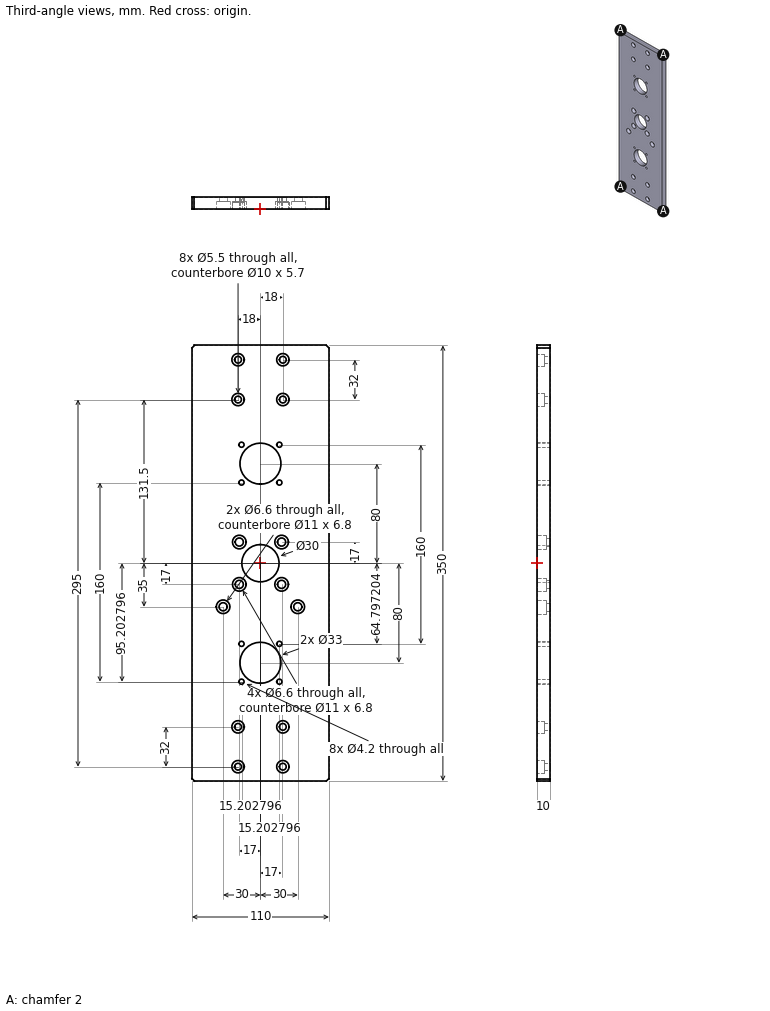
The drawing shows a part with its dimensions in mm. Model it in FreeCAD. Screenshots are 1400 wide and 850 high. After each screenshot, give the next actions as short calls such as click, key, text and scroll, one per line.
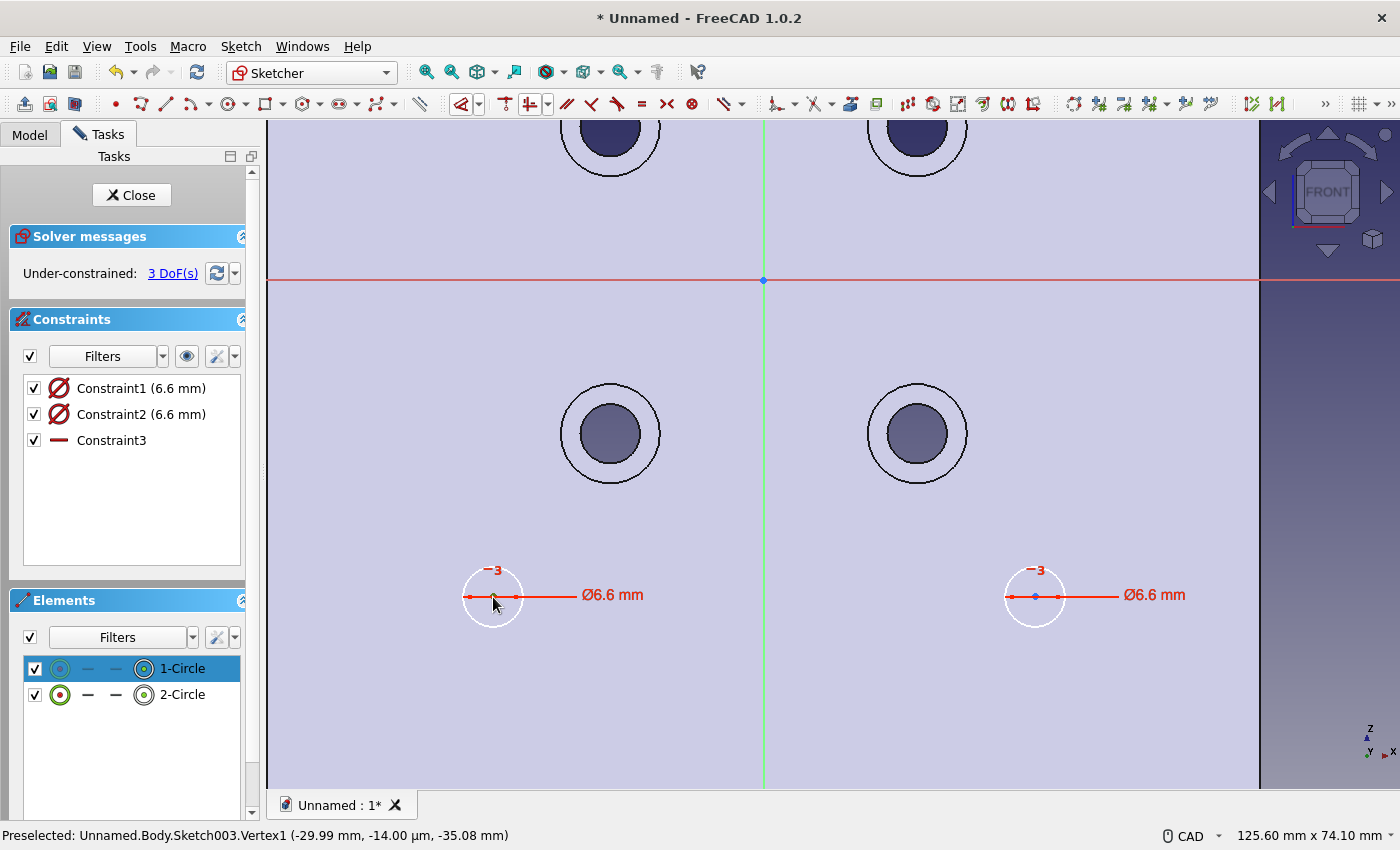
key(l)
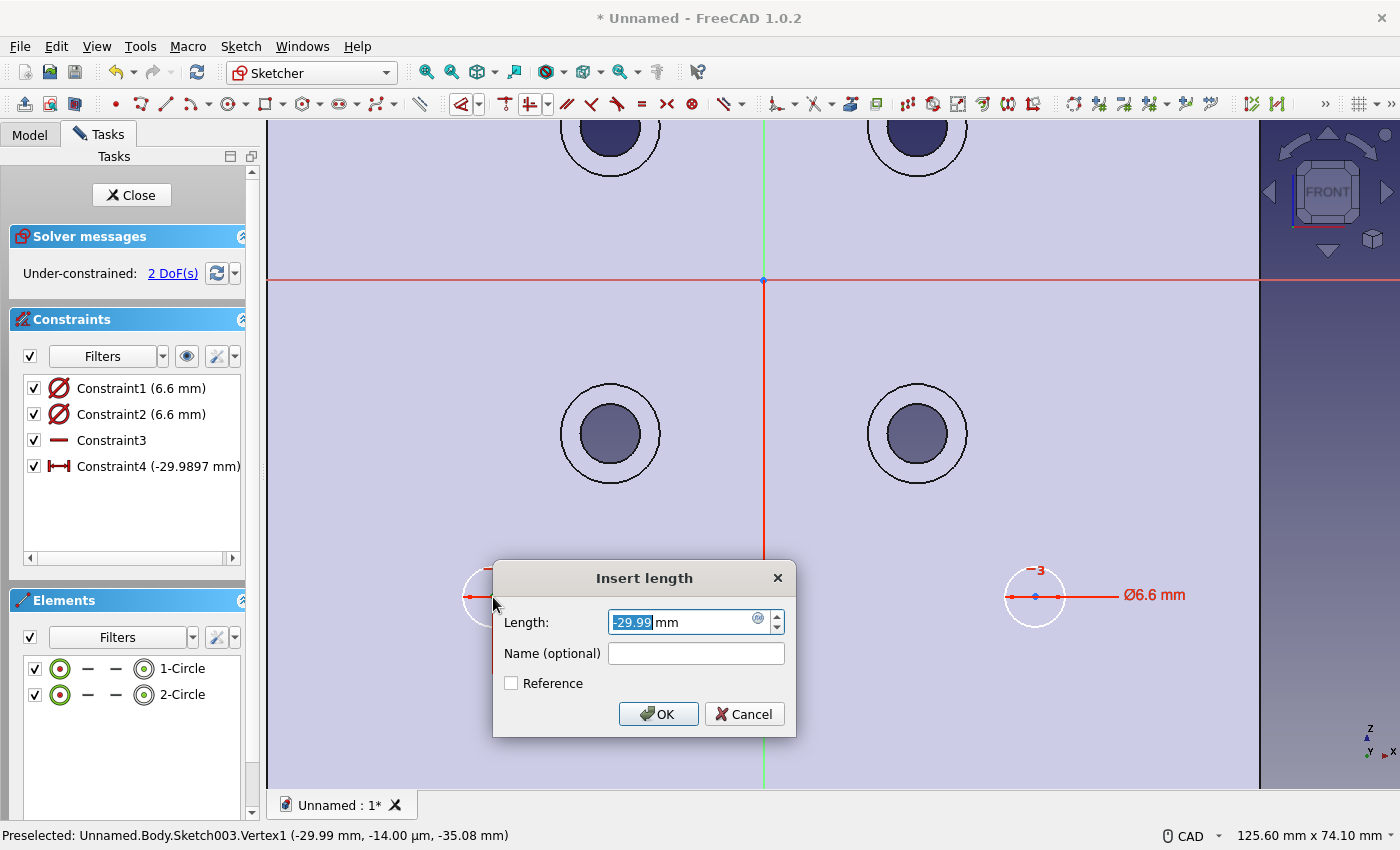
text(-30)
key(Return)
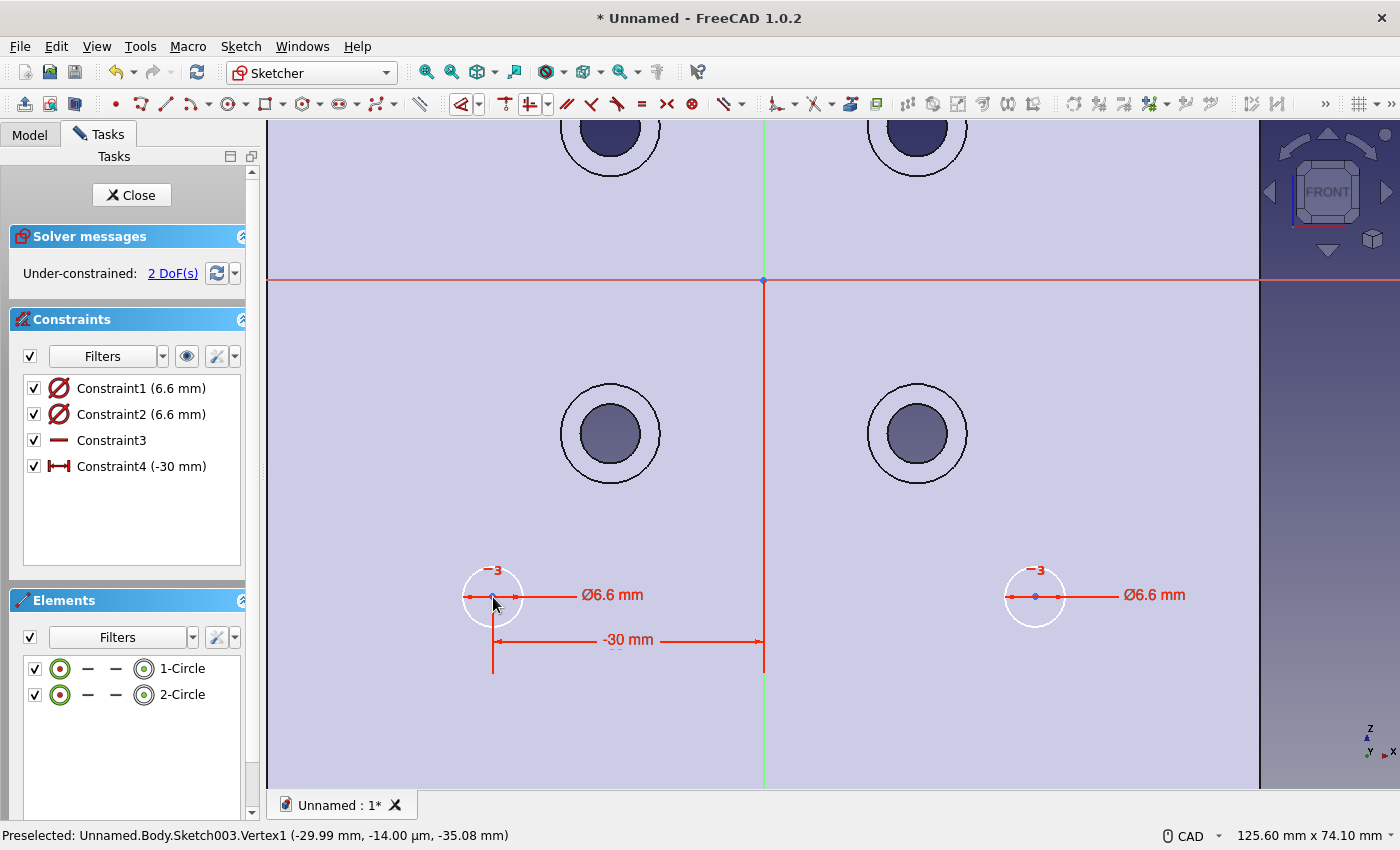
click(493, 597)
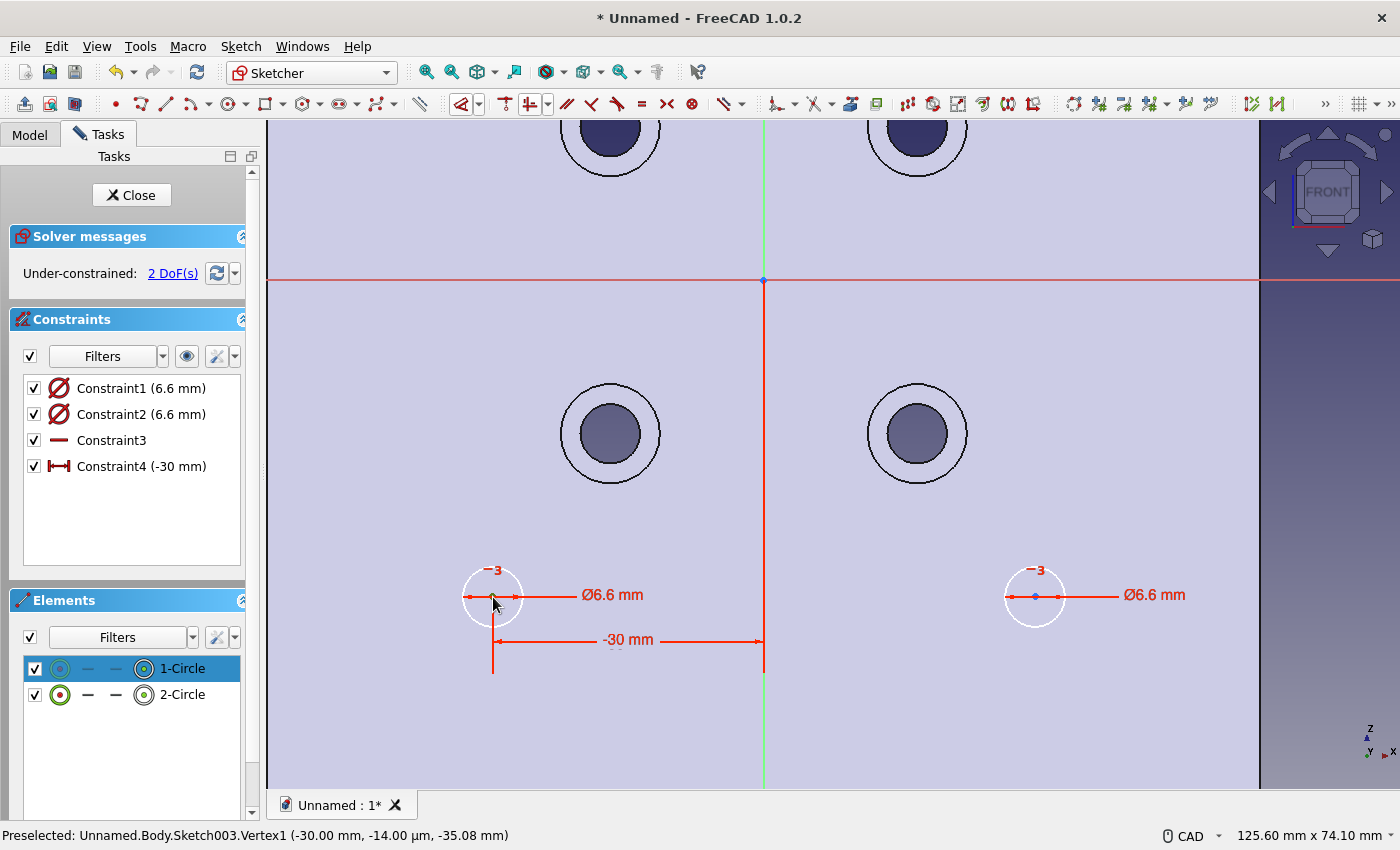
click(478, 104)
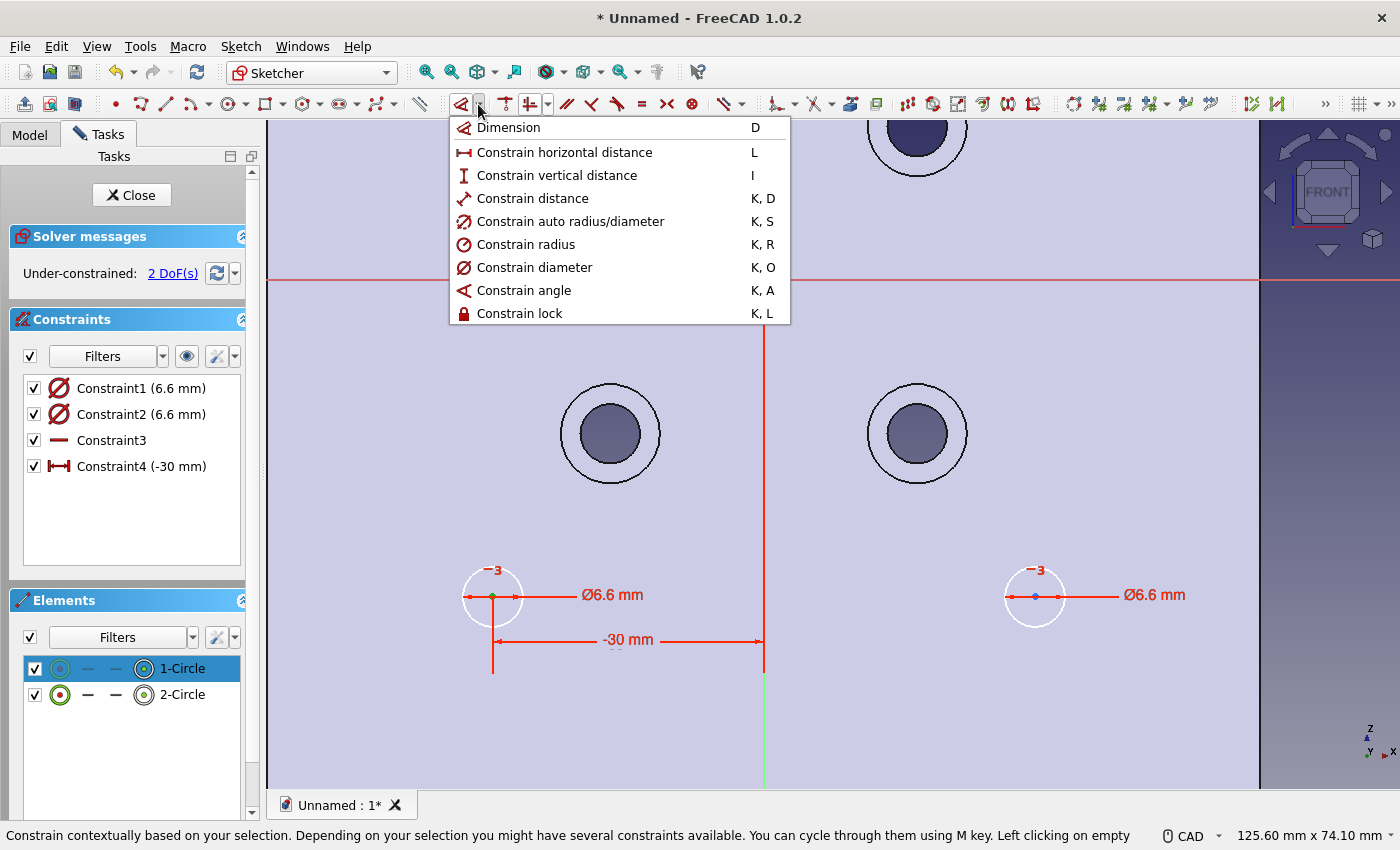
click(620, 176)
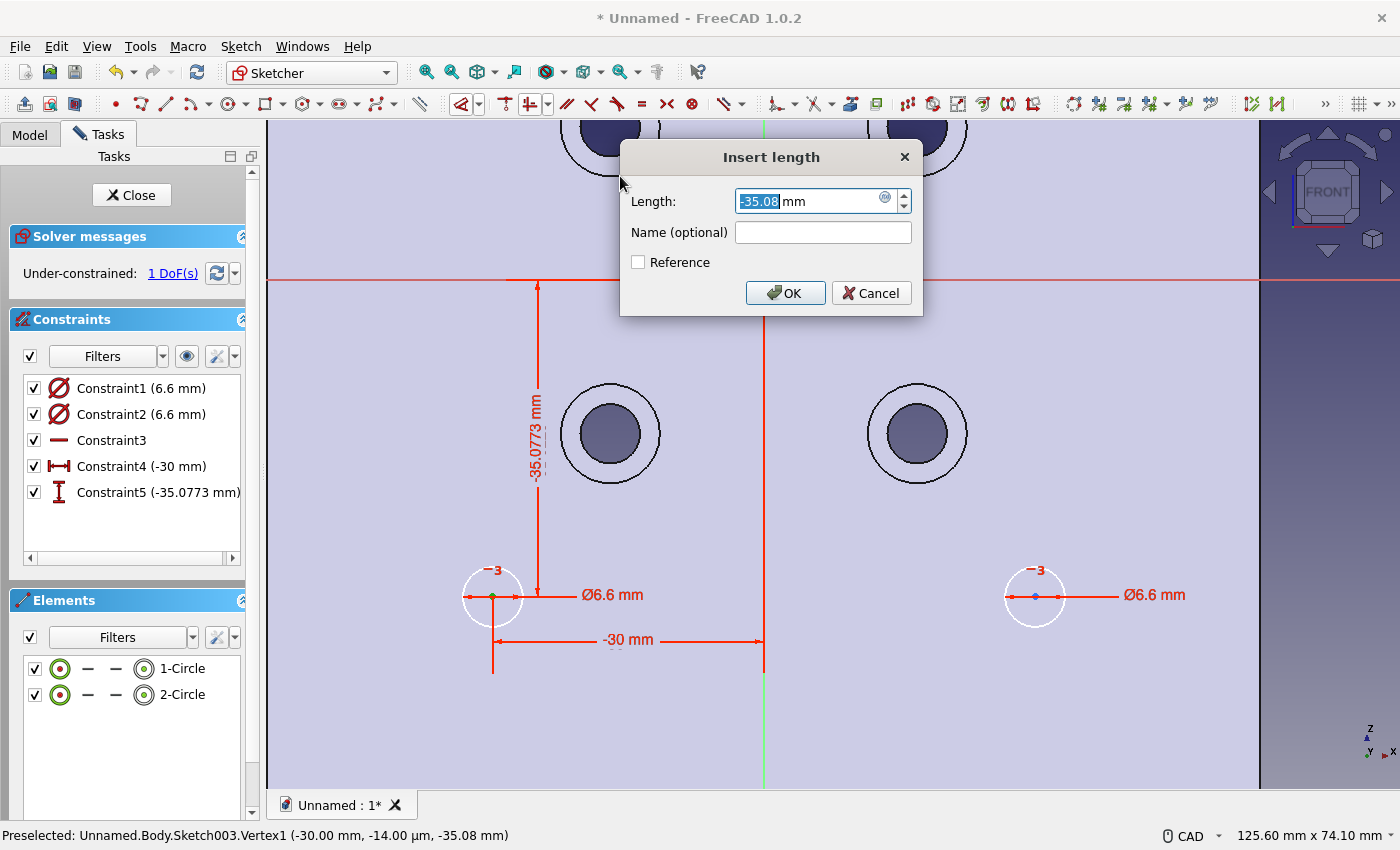
text(-35)
key(Return)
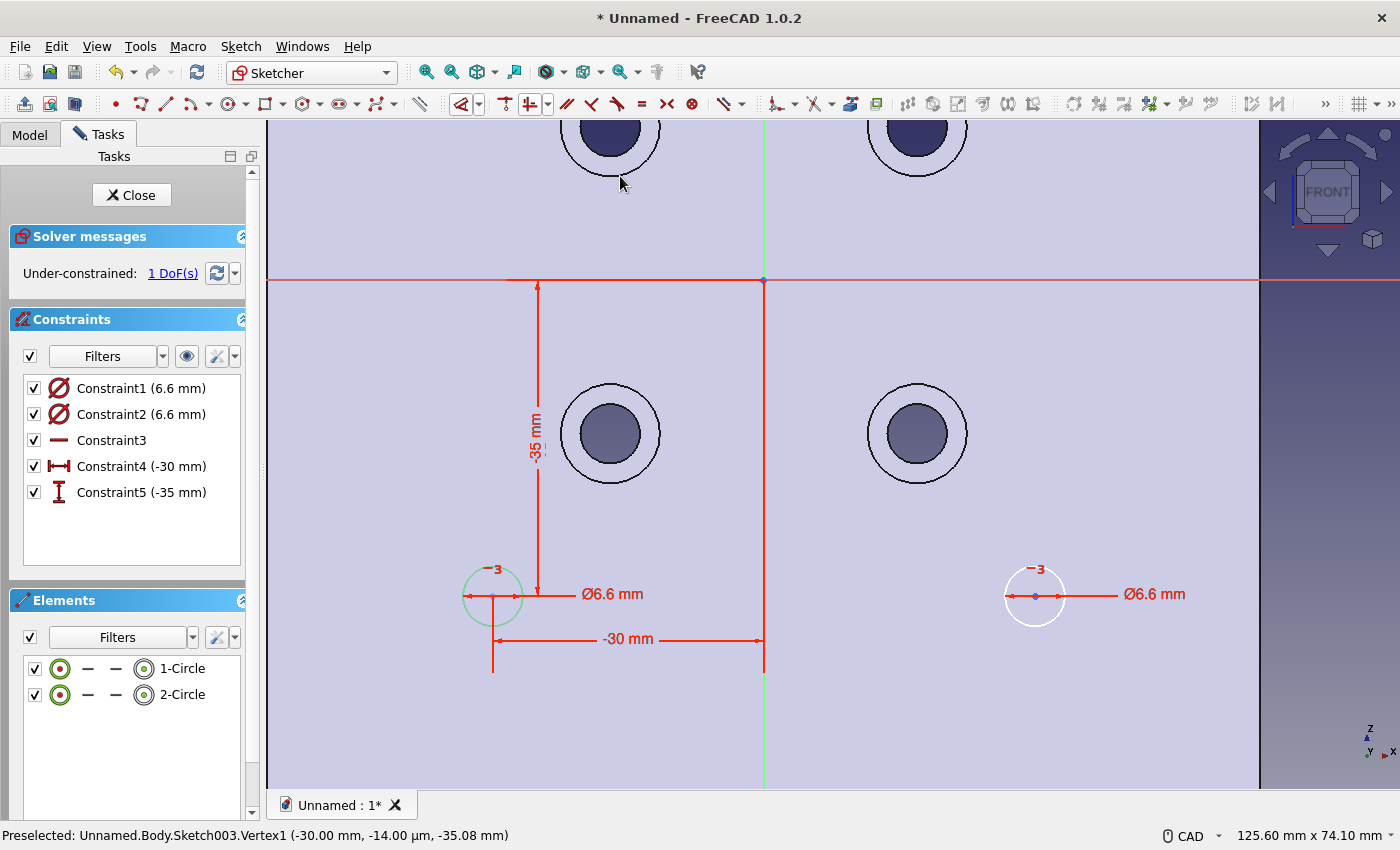
click(1035, 596)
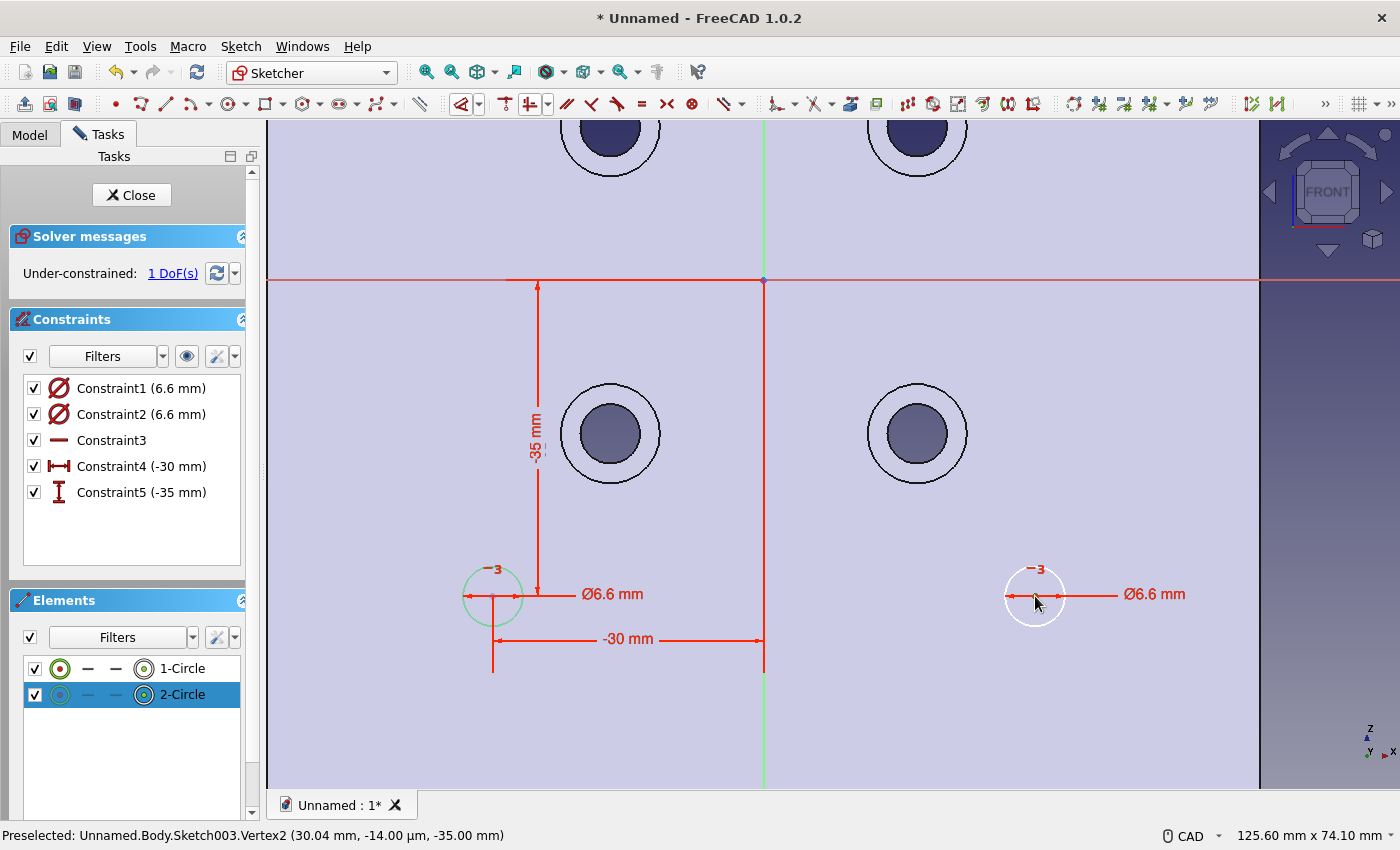
key(l)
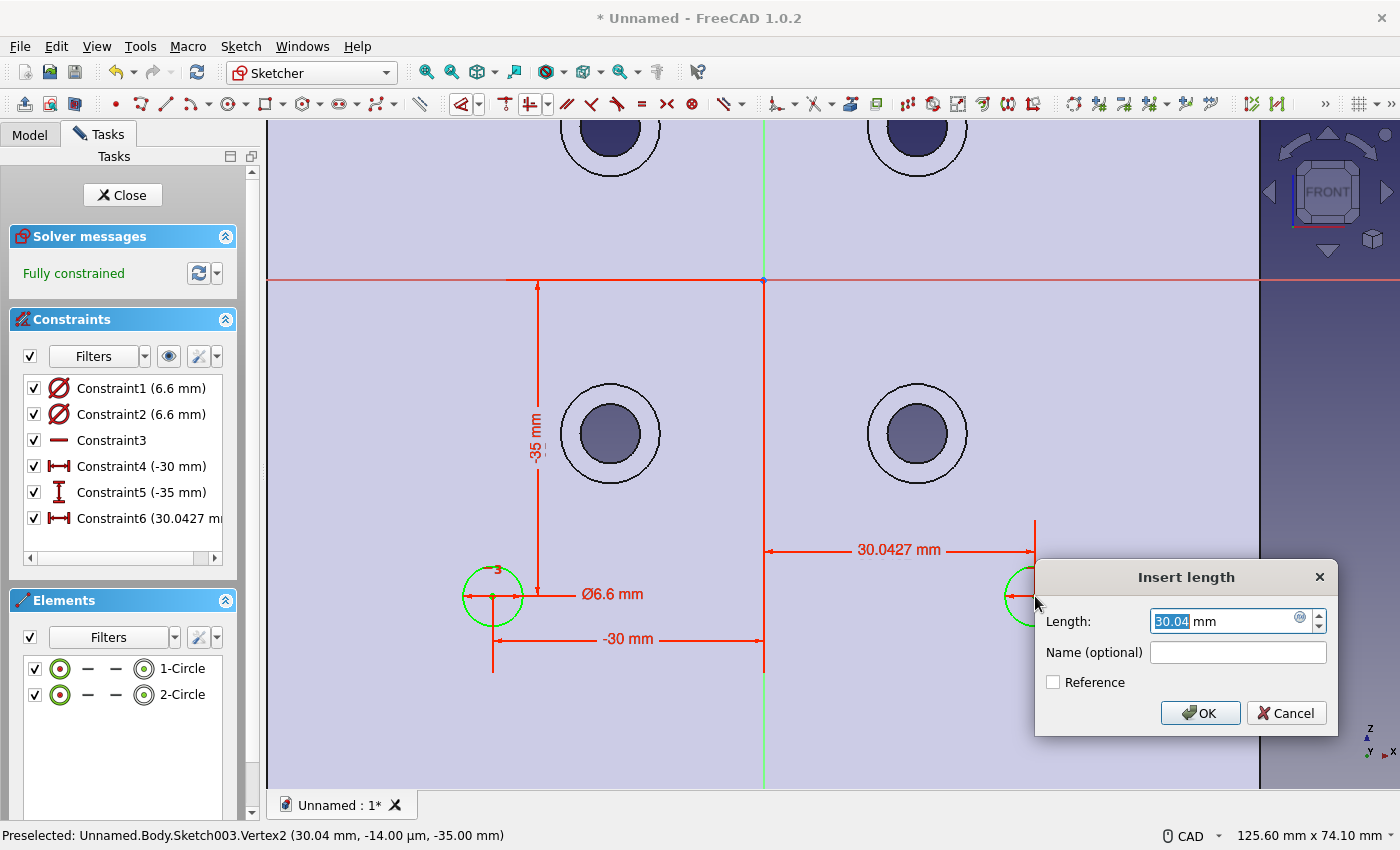
text(30)
key(Return)